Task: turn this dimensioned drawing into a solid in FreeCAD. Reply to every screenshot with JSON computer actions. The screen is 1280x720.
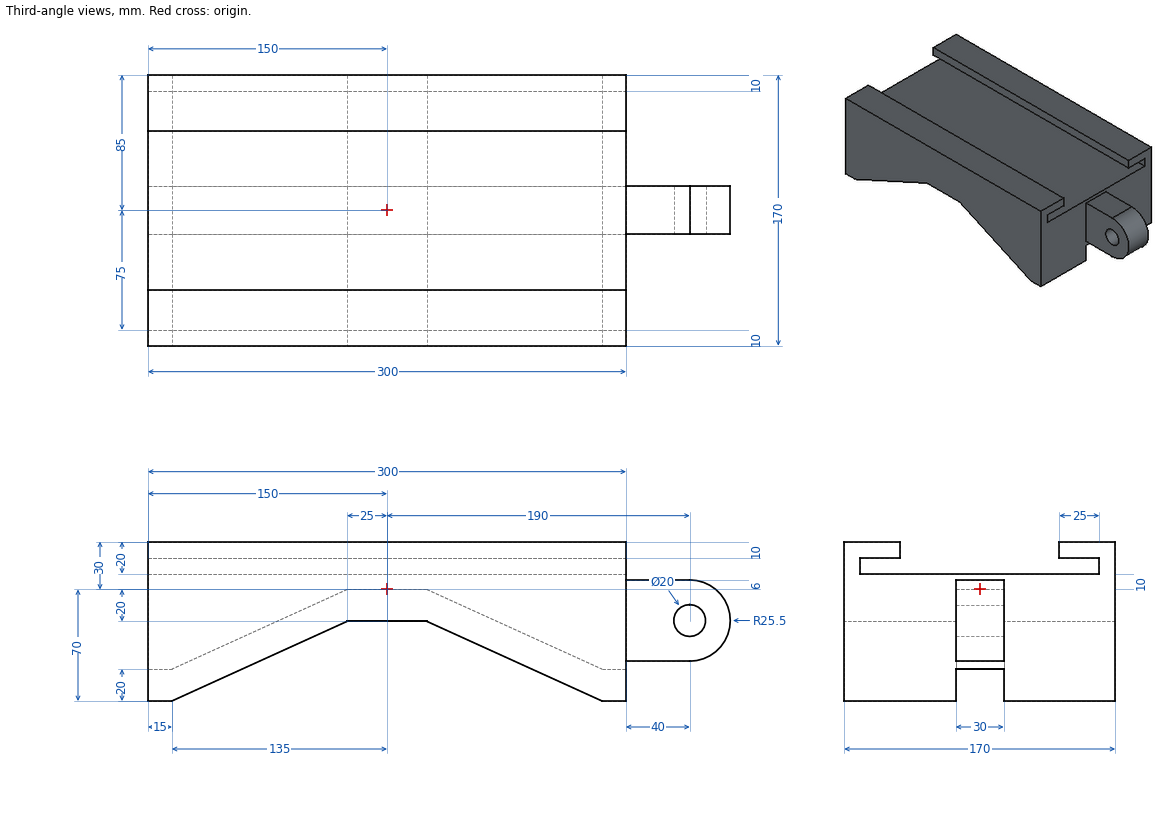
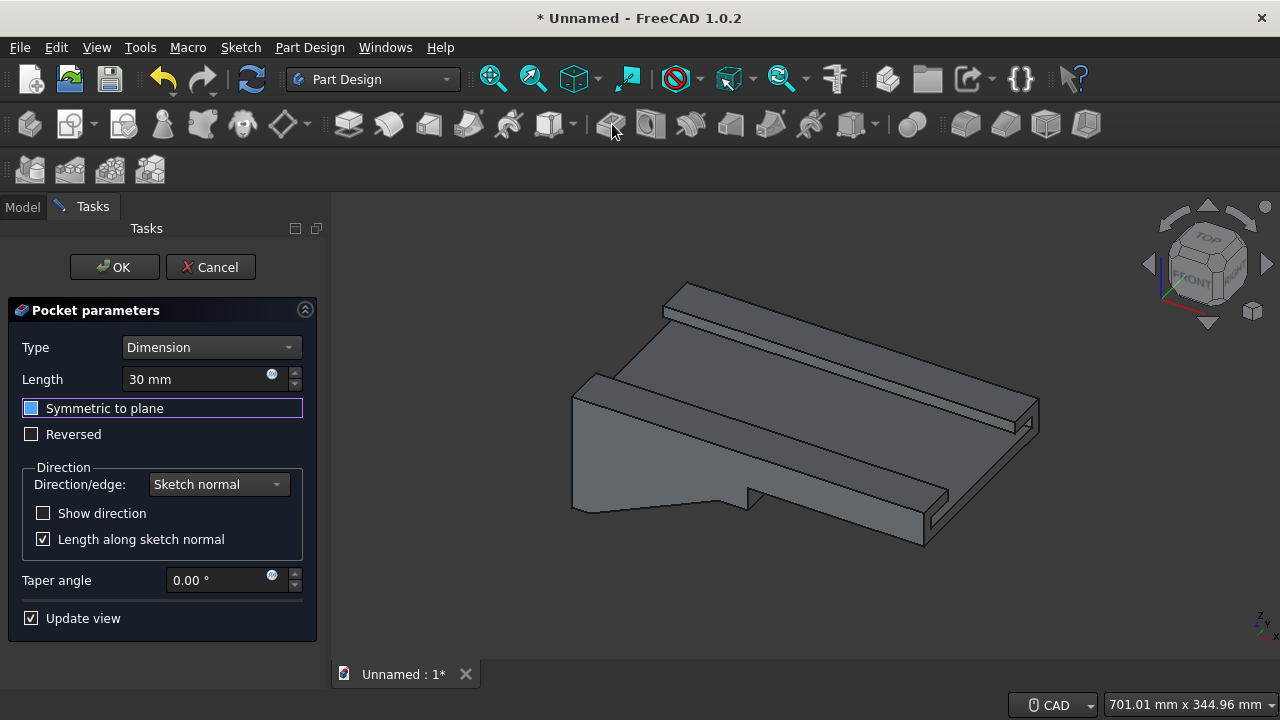
{"action": "left_click", "coordinate": [30, 408]}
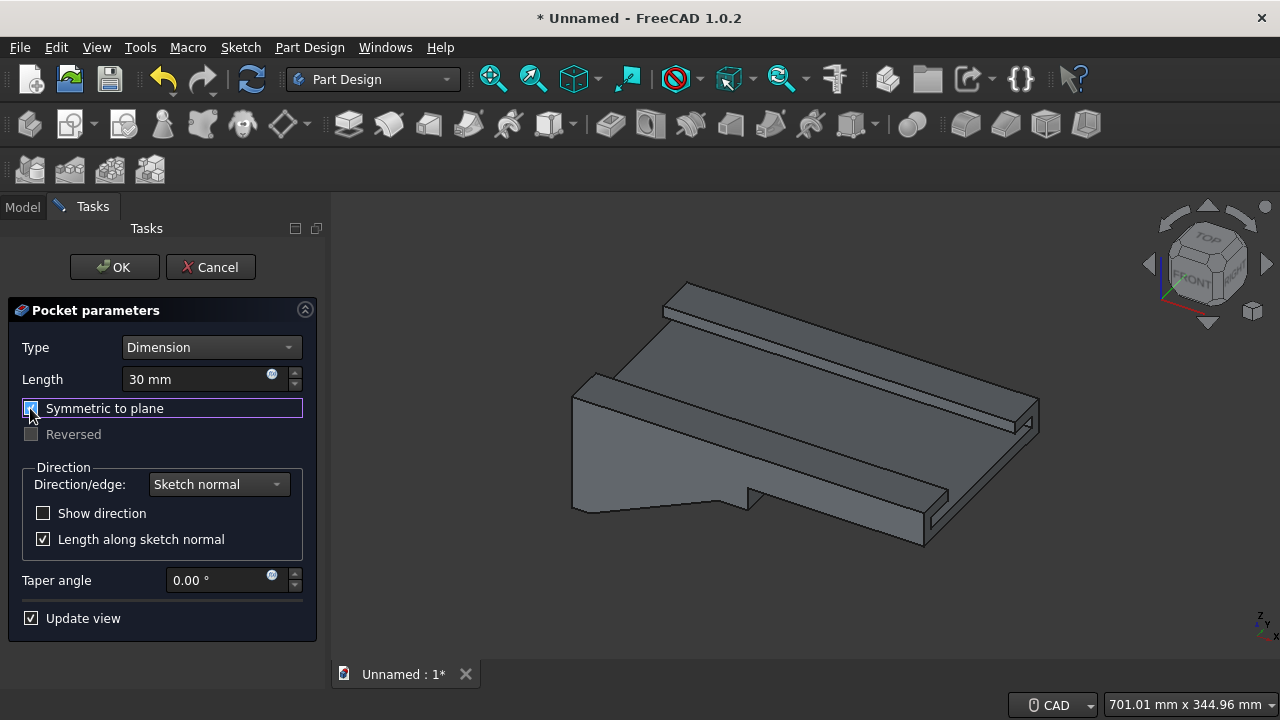
{"action": "left_click", "coordinate": [115, 267]}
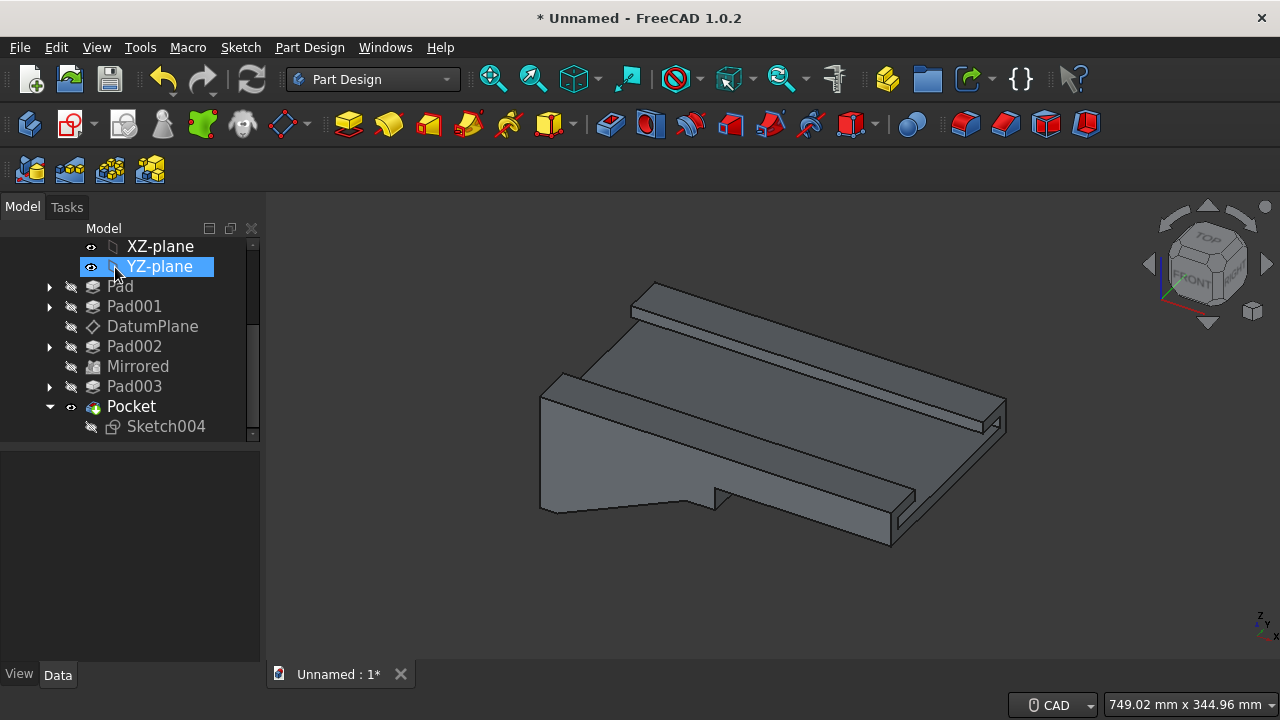
{"action": "left_click", "coordinate": [116, 387]}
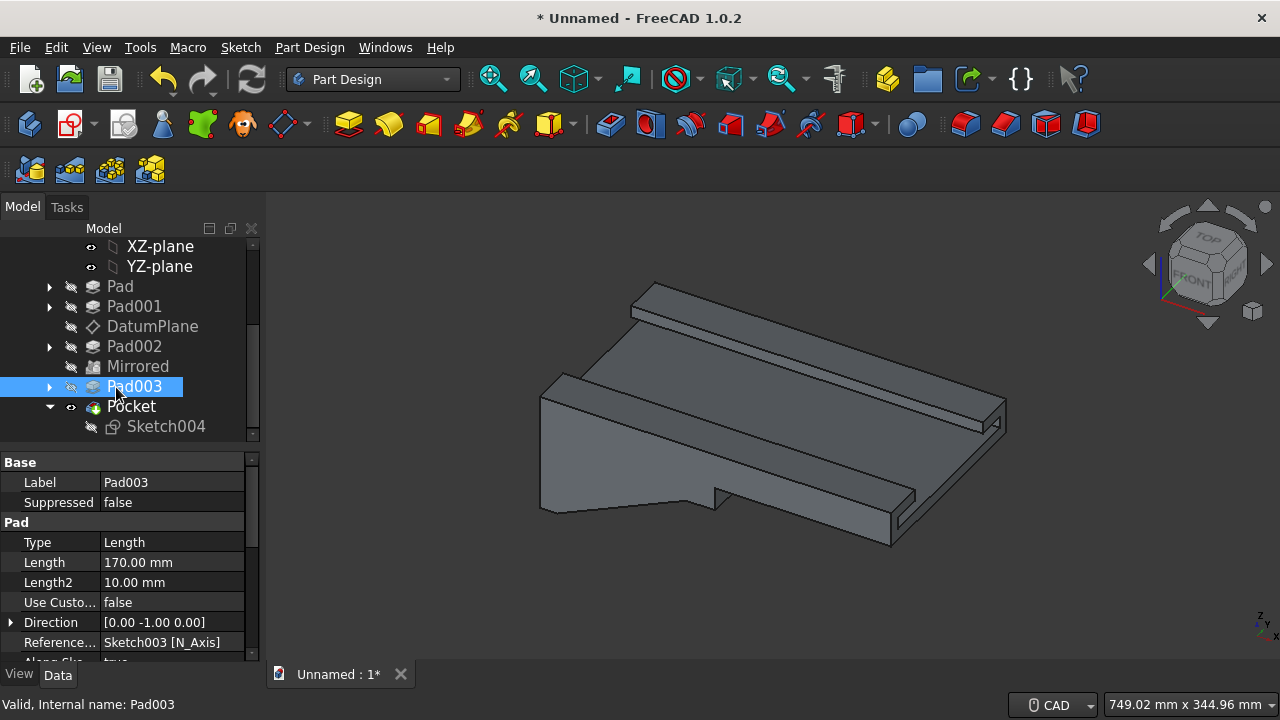
{"action": "left_click", "coordinate": [116, 407], "text": "ctrl"}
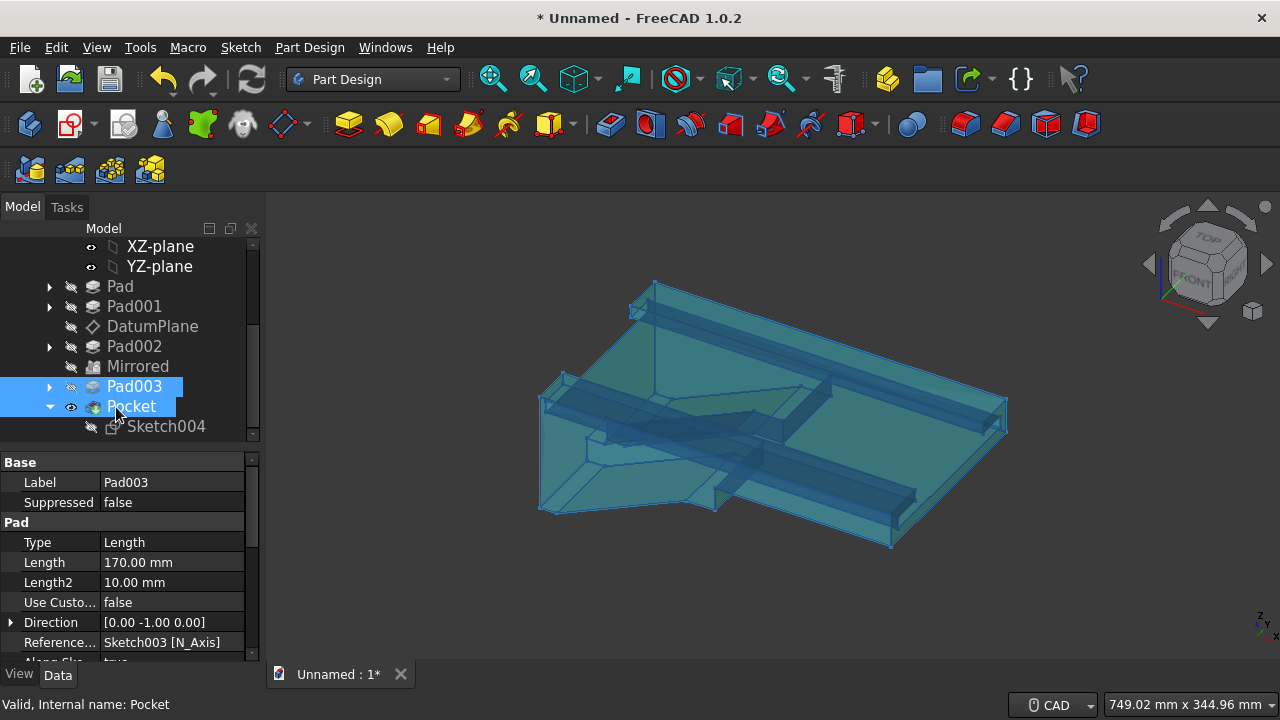
{"action": "left_click", "coordinate": [30, 170]}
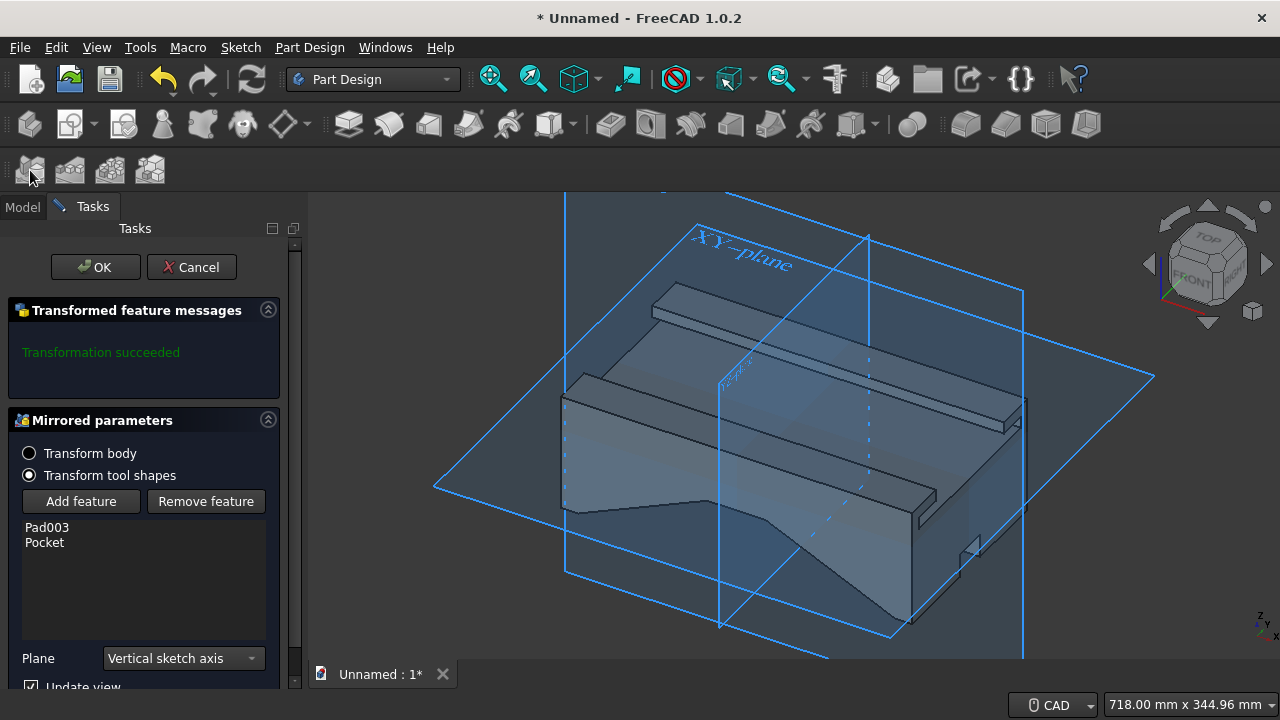
{"action": "left_click", "coordinate": [184, 658]}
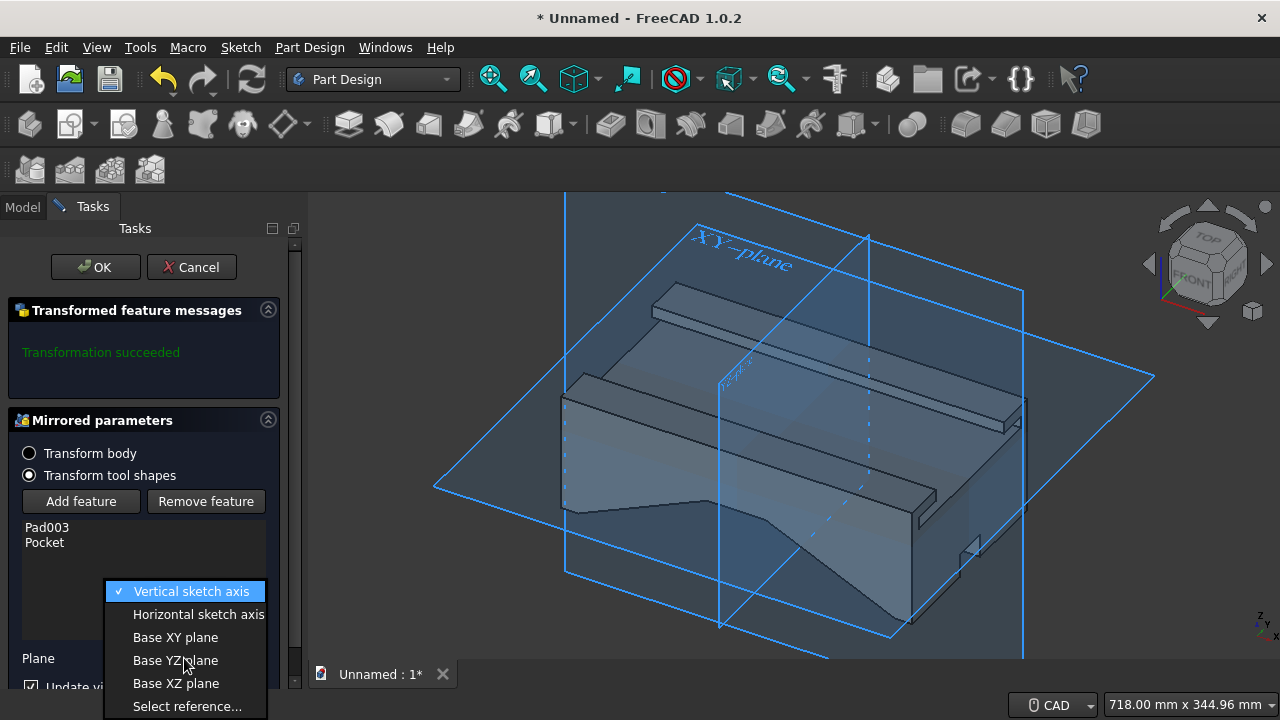
{"action": "left_click", "coordinate": [184, 660]}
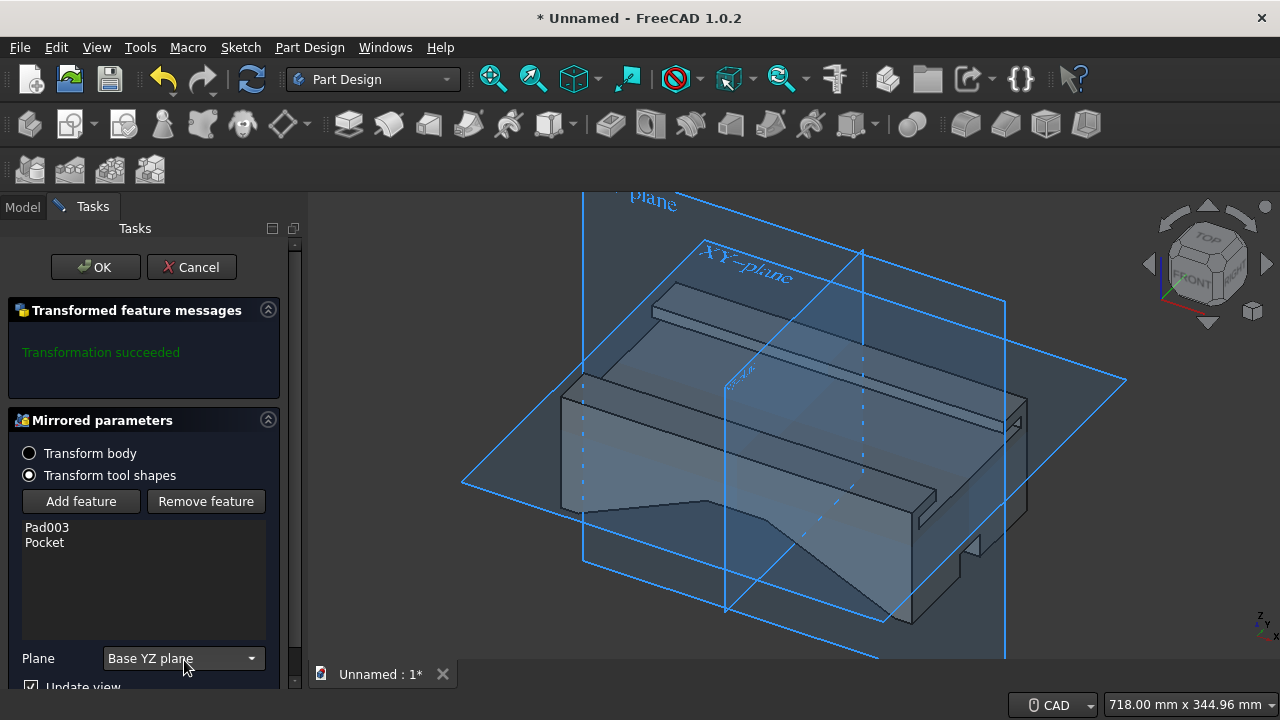
{"action": "left_click", "coordinate": [96, 267]}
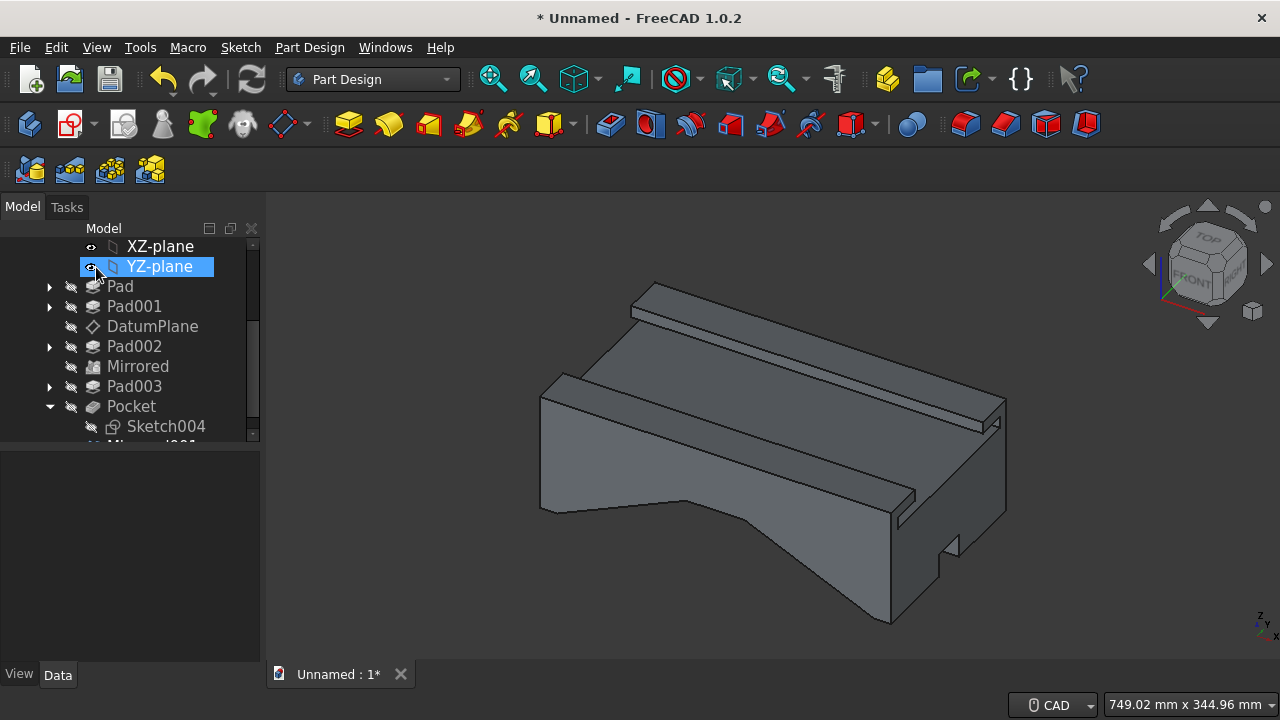
{"action": "left_click", "coordinate": [70, 124]}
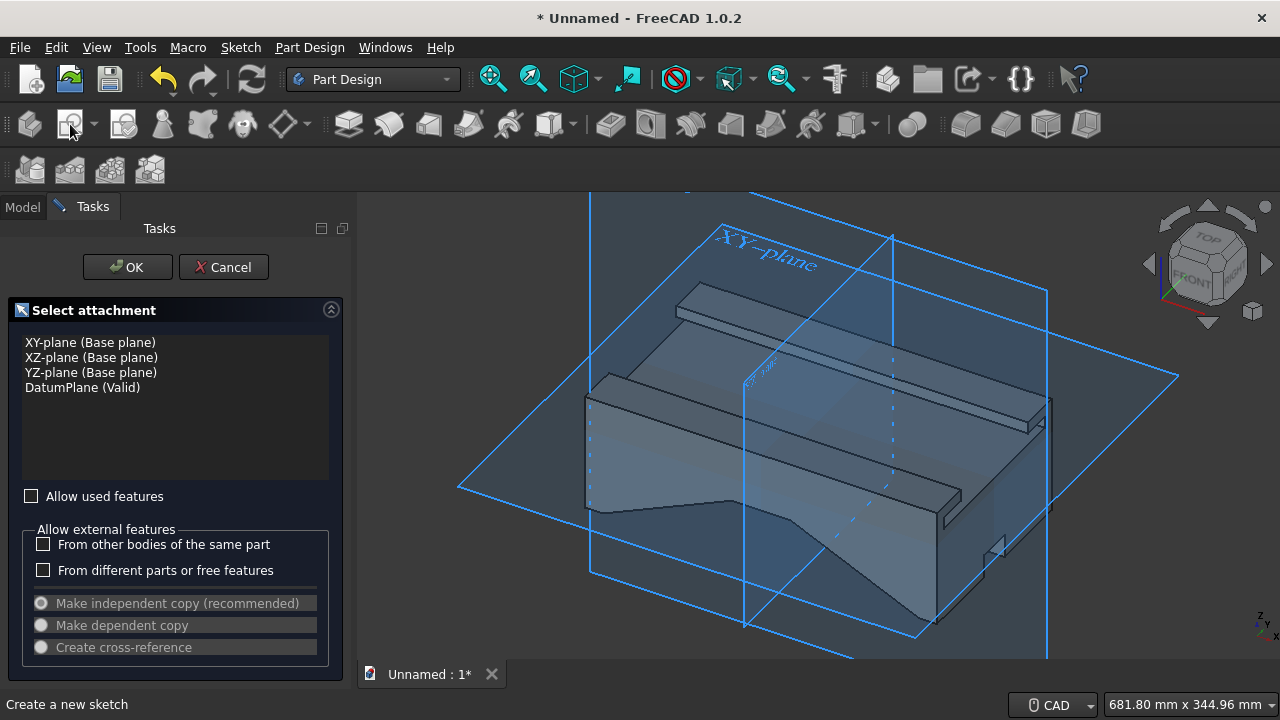
{"action": "left_click", "coordinate": [82, 358]}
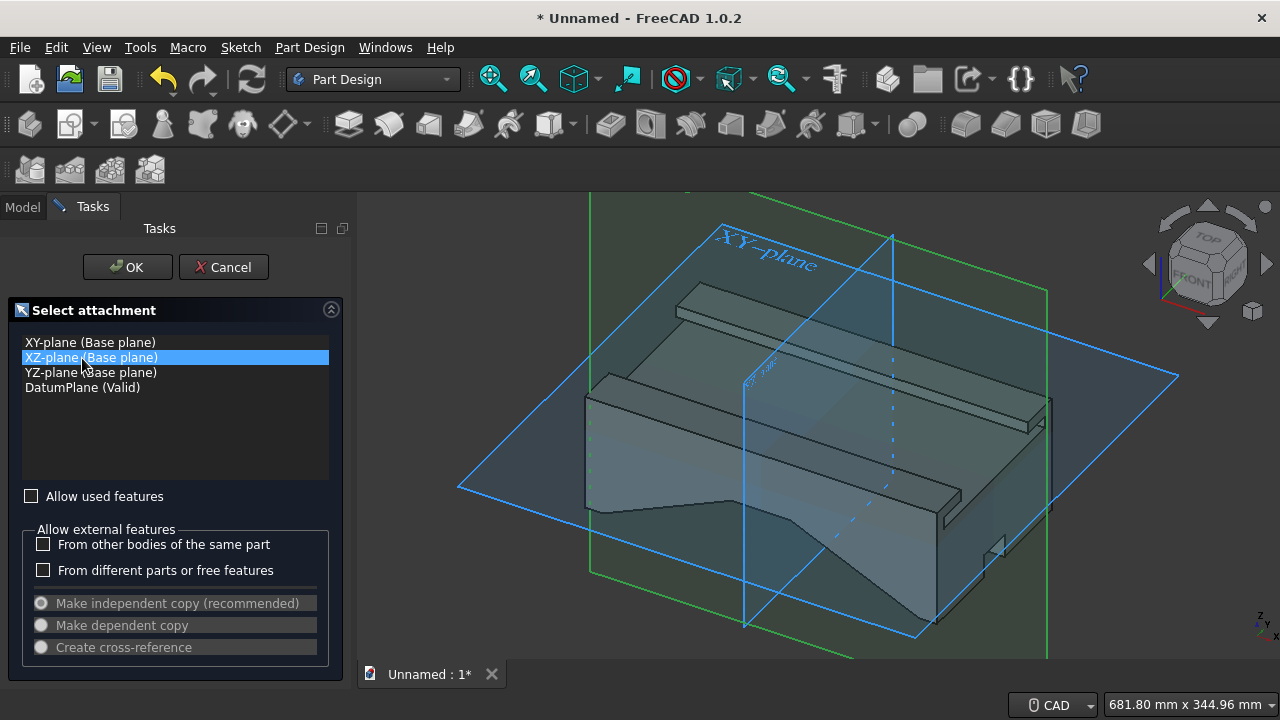
{"action": "left_click", "coordinate": [128, 267]}